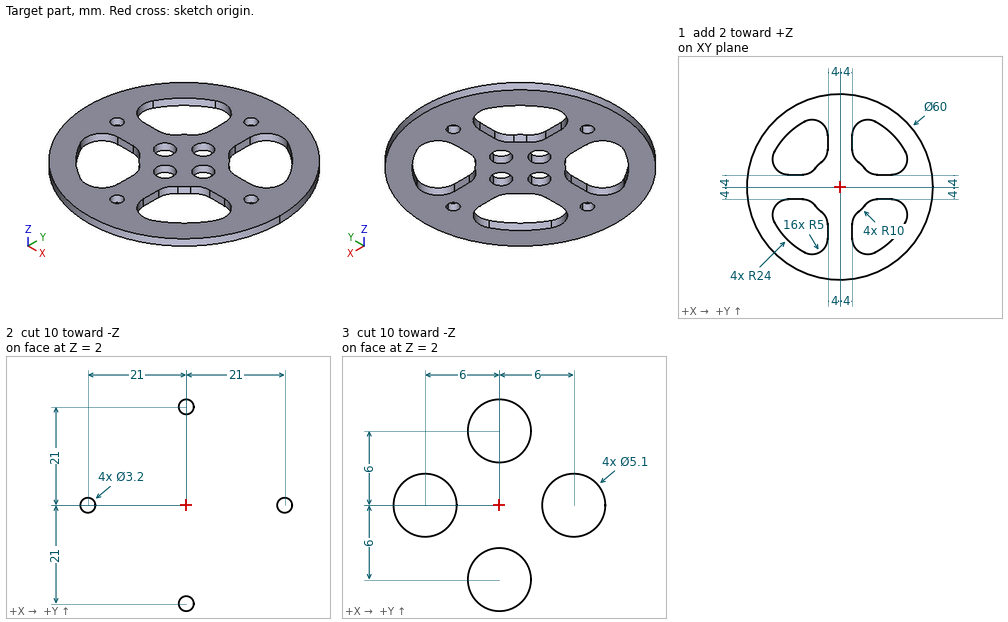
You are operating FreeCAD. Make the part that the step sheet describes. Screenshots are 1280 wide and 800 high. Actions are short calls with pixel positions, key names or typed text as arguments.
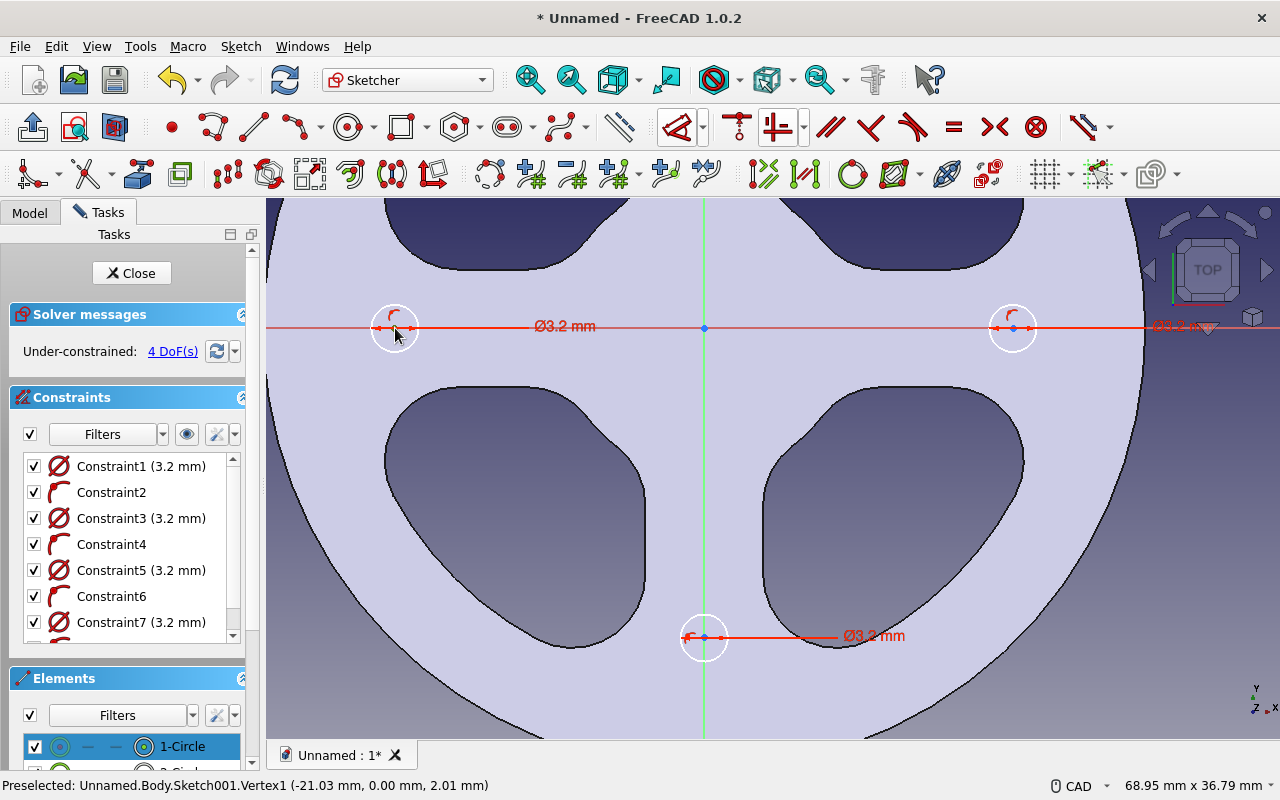
key(l)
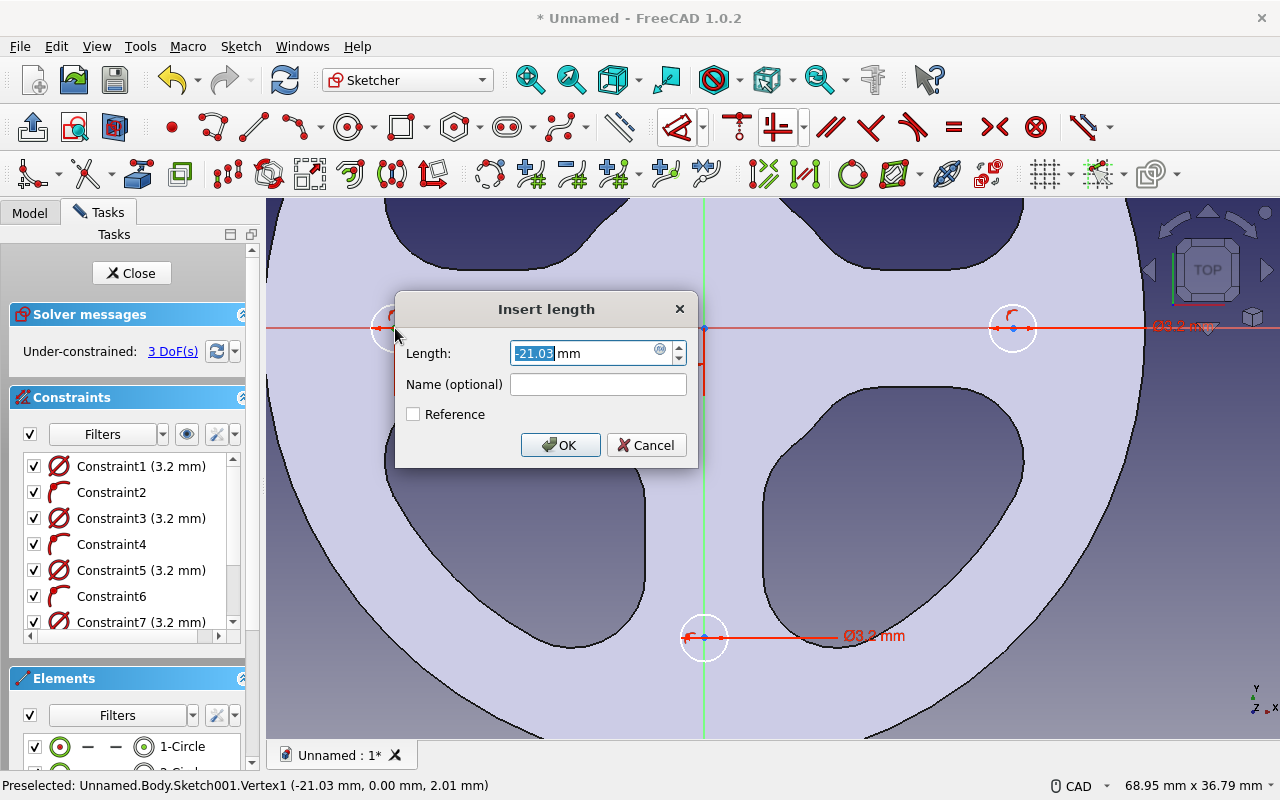
text(-21)
key(Return)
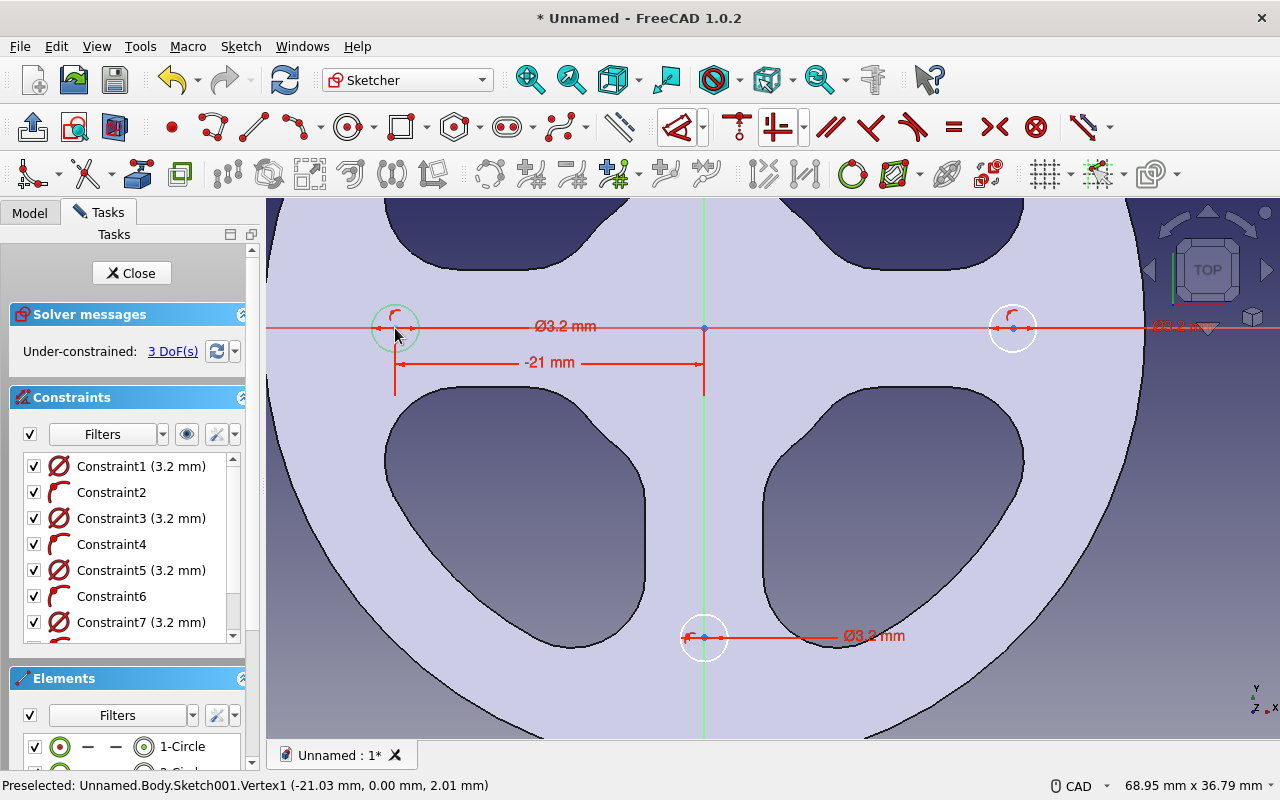
scroll(705, 639, down, 3)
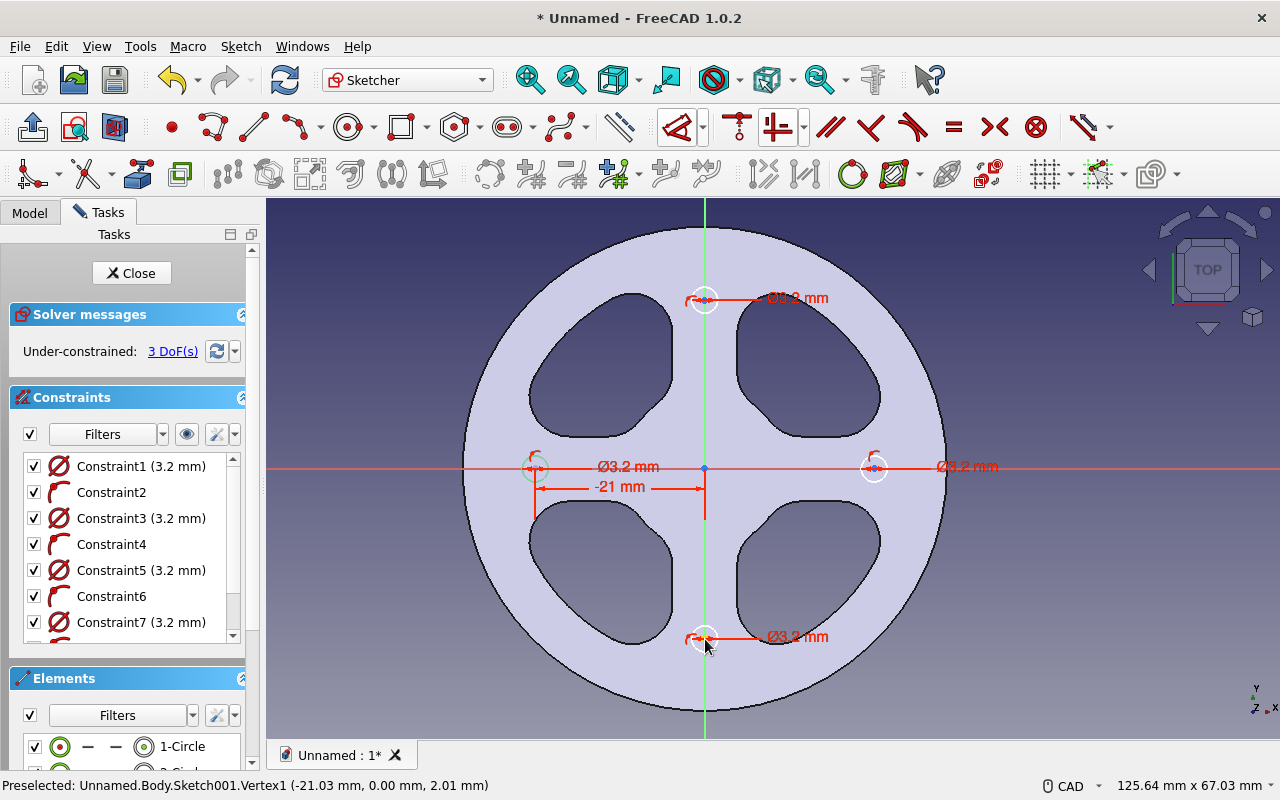
click(705, 300)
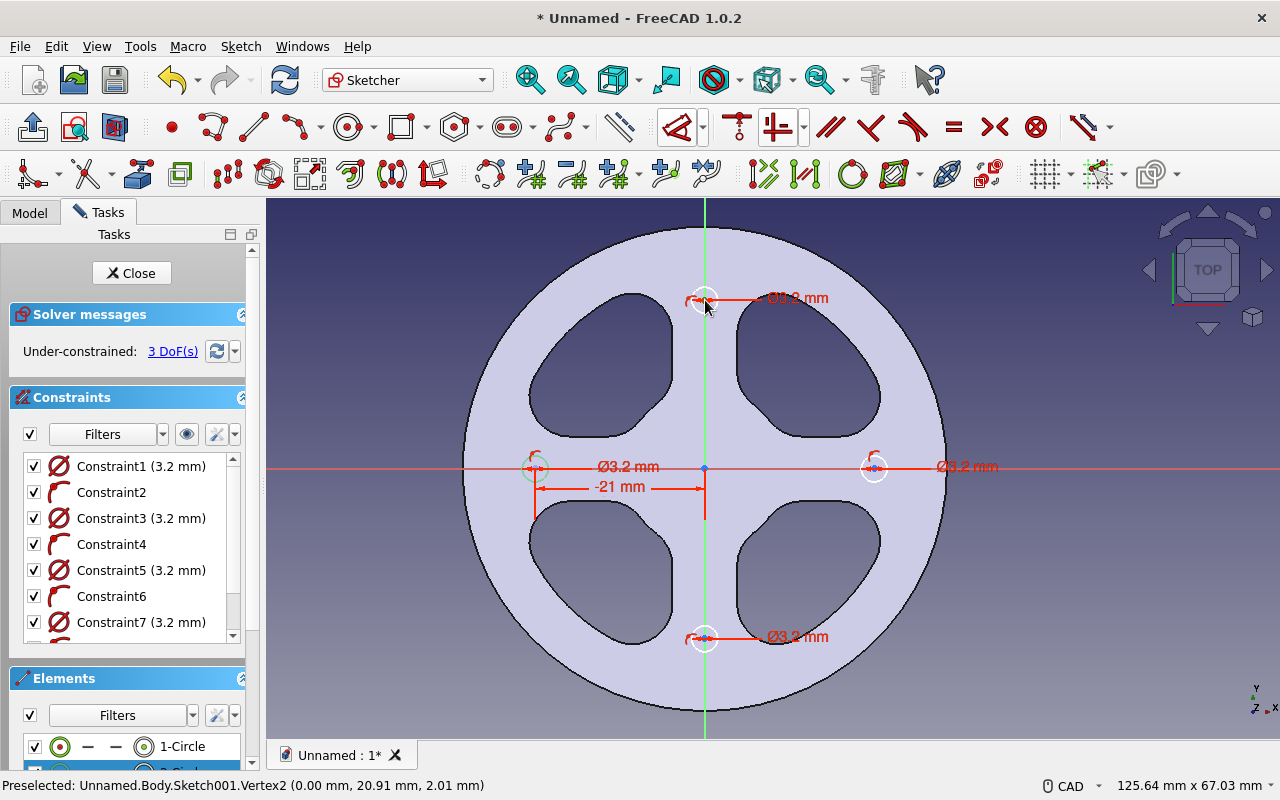
key(i)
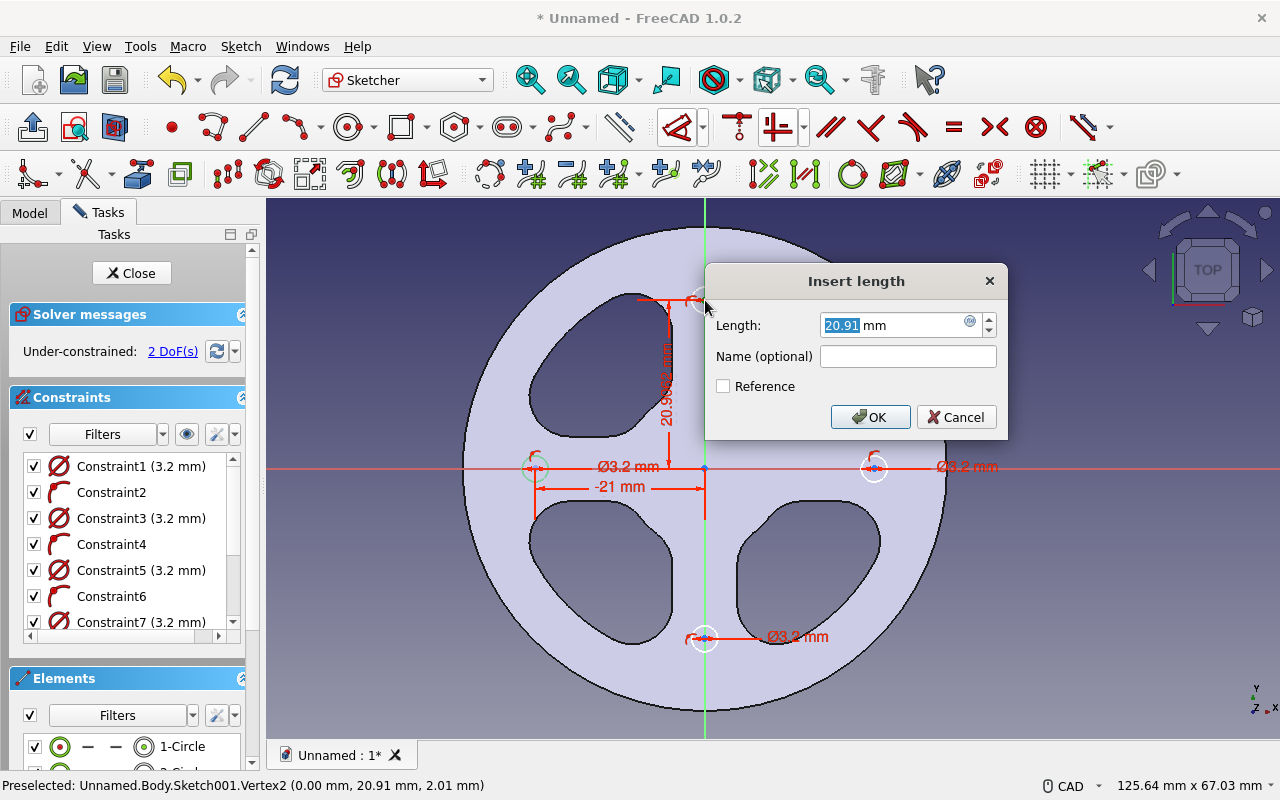
text(21)
key(Return)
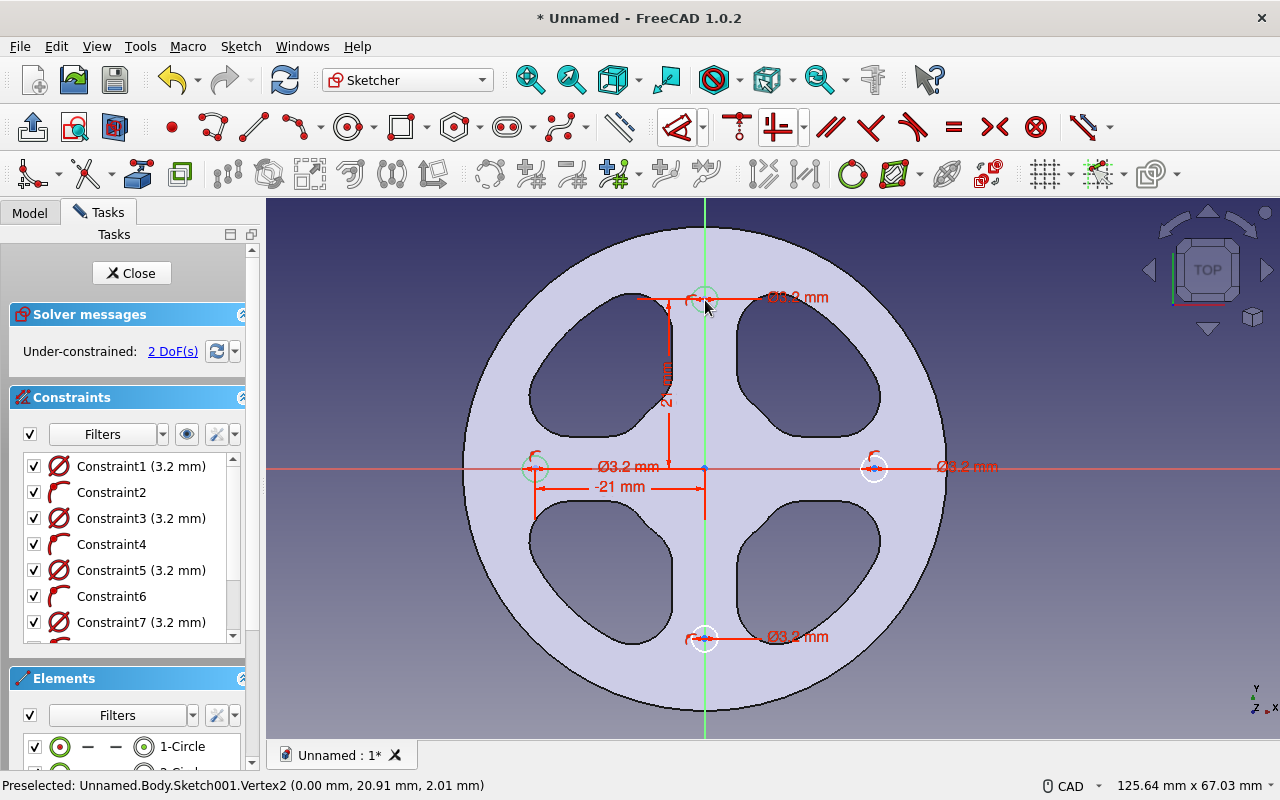
click(874, 469)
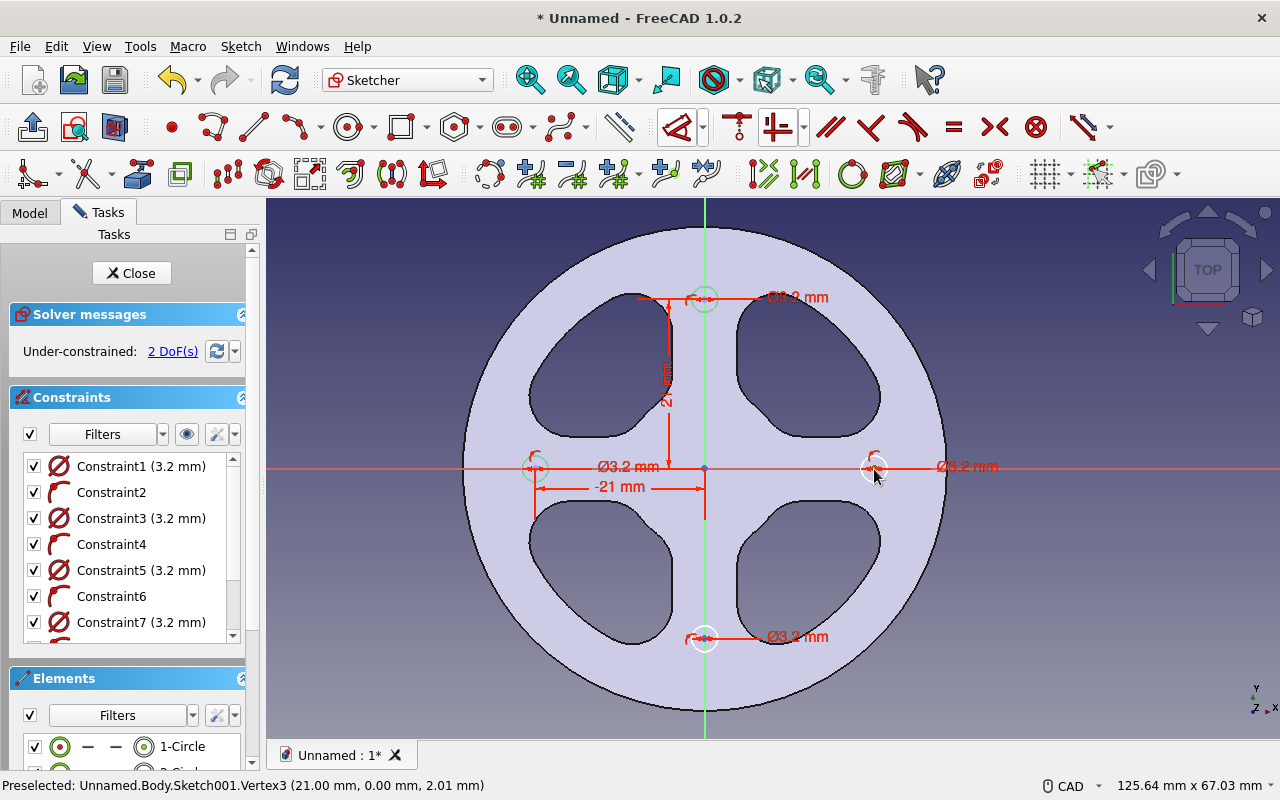
click(702, 128)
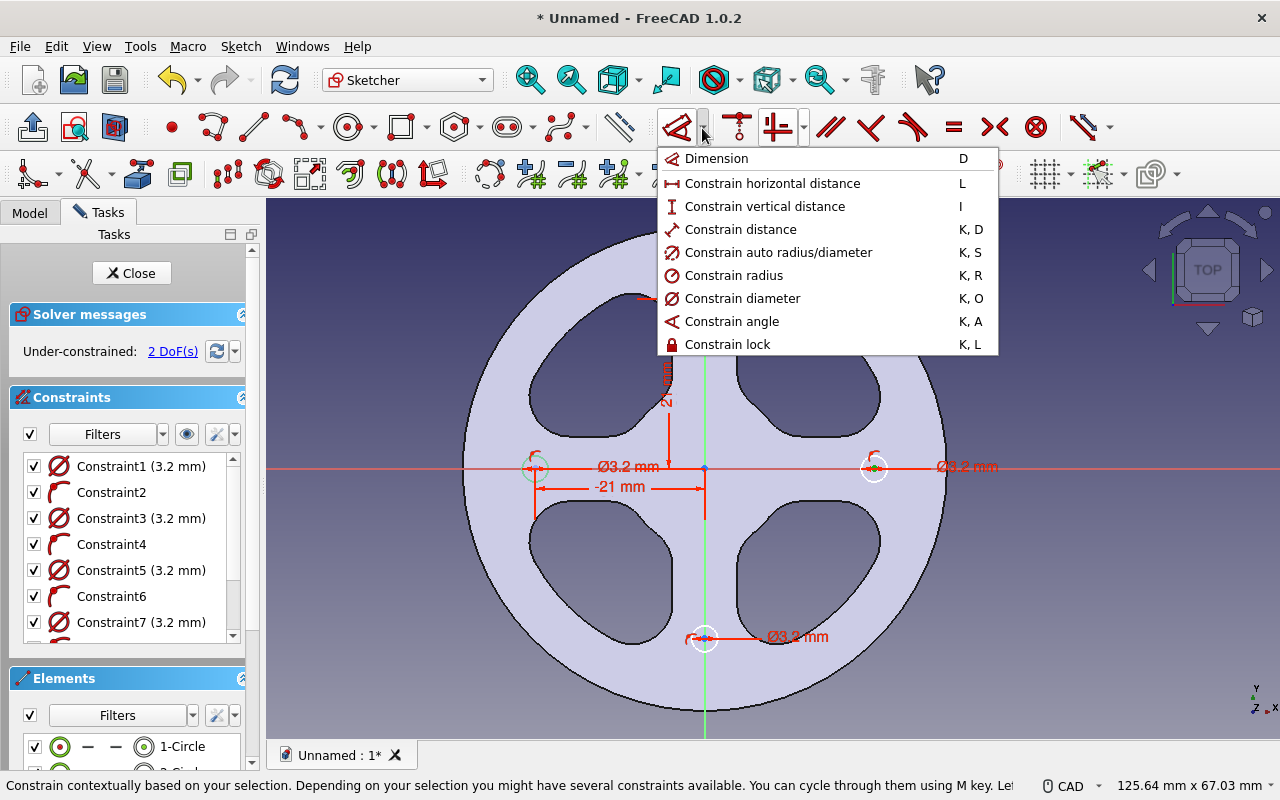
click(828, 184)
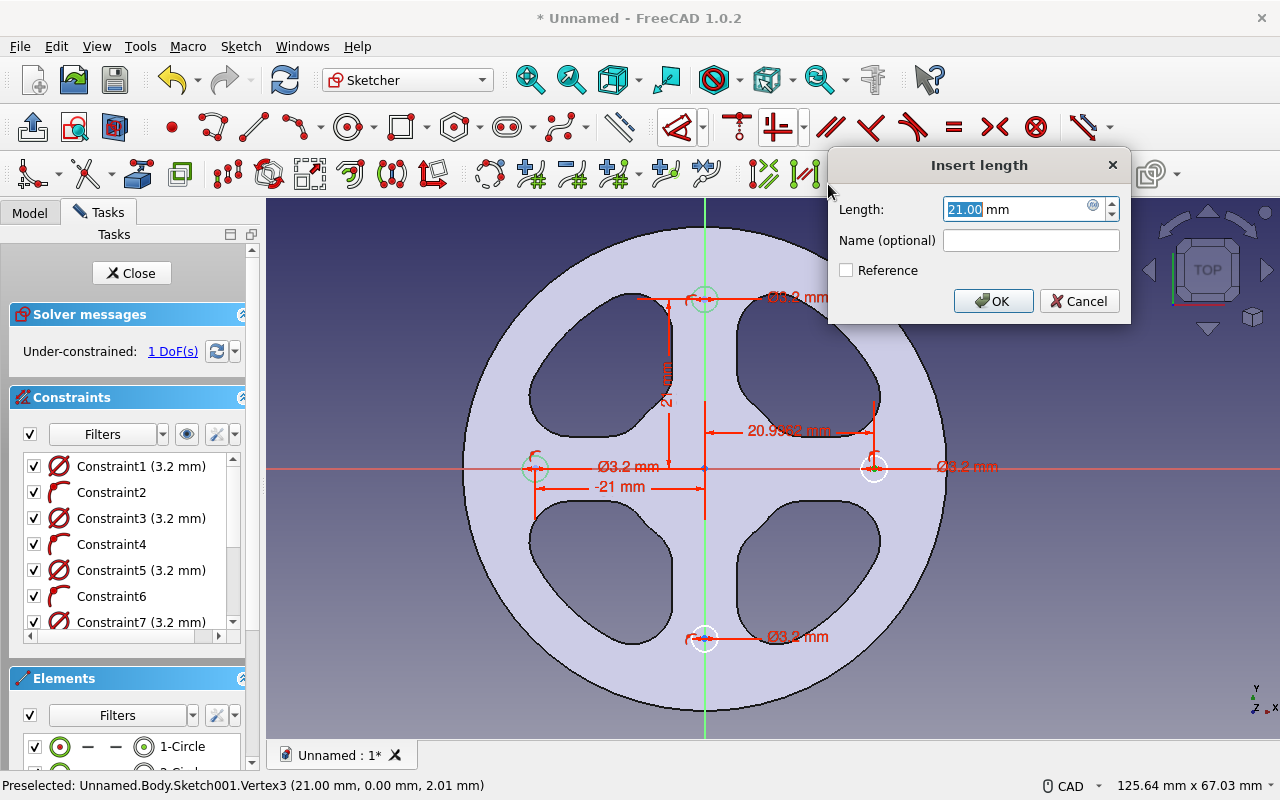
text(21)
key(Return)